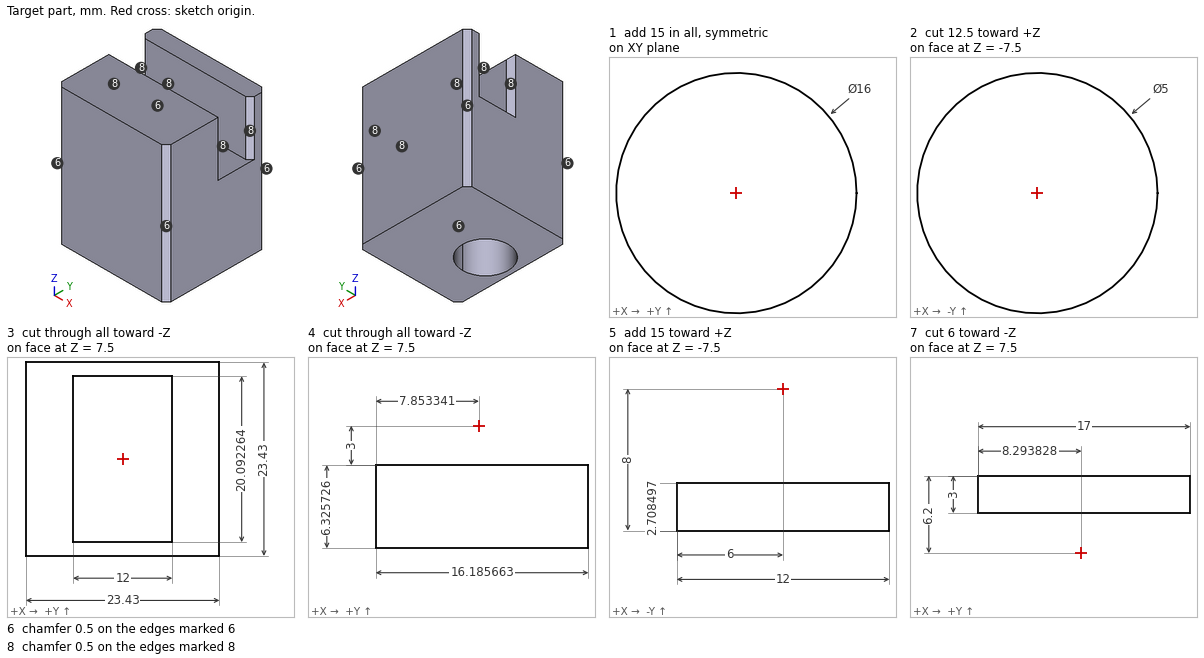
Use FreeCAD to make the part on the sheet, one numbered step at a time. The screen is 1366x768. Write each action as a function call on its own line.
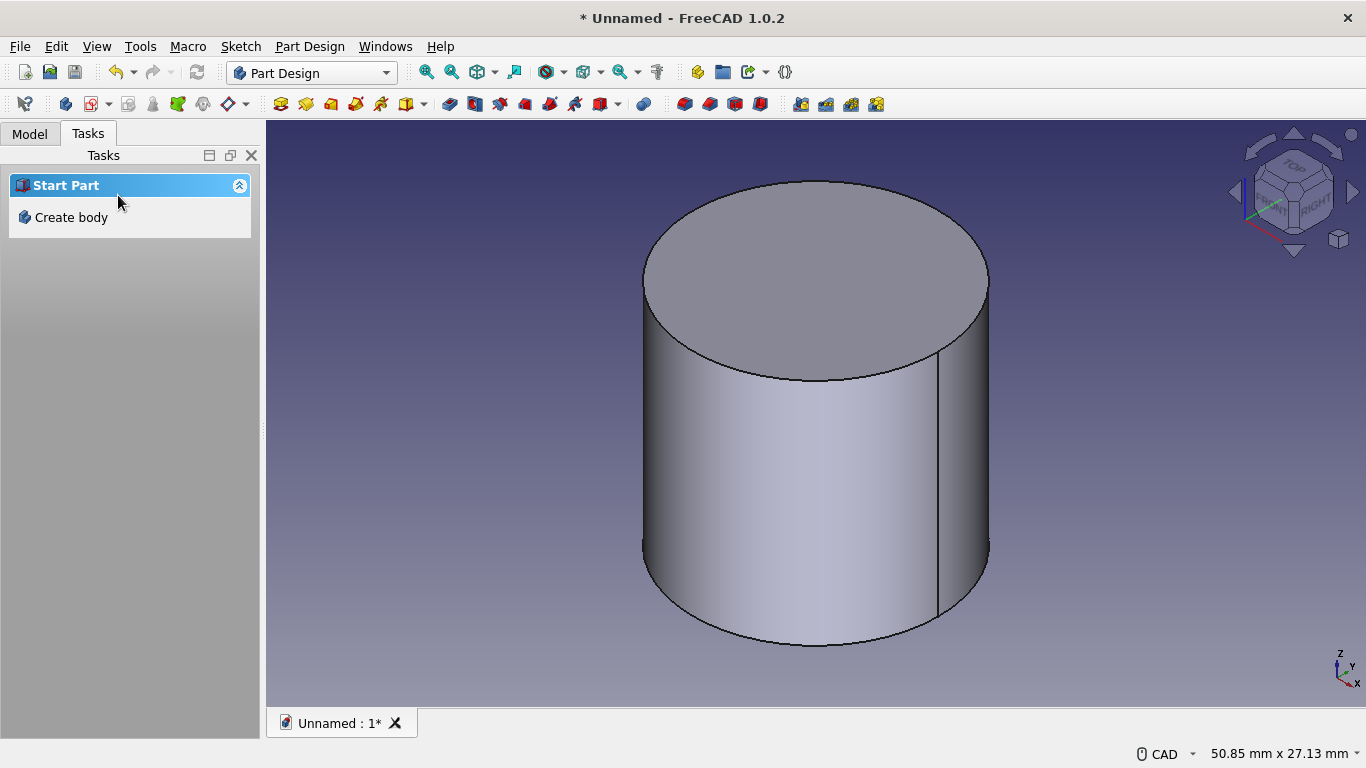
click(816, 280)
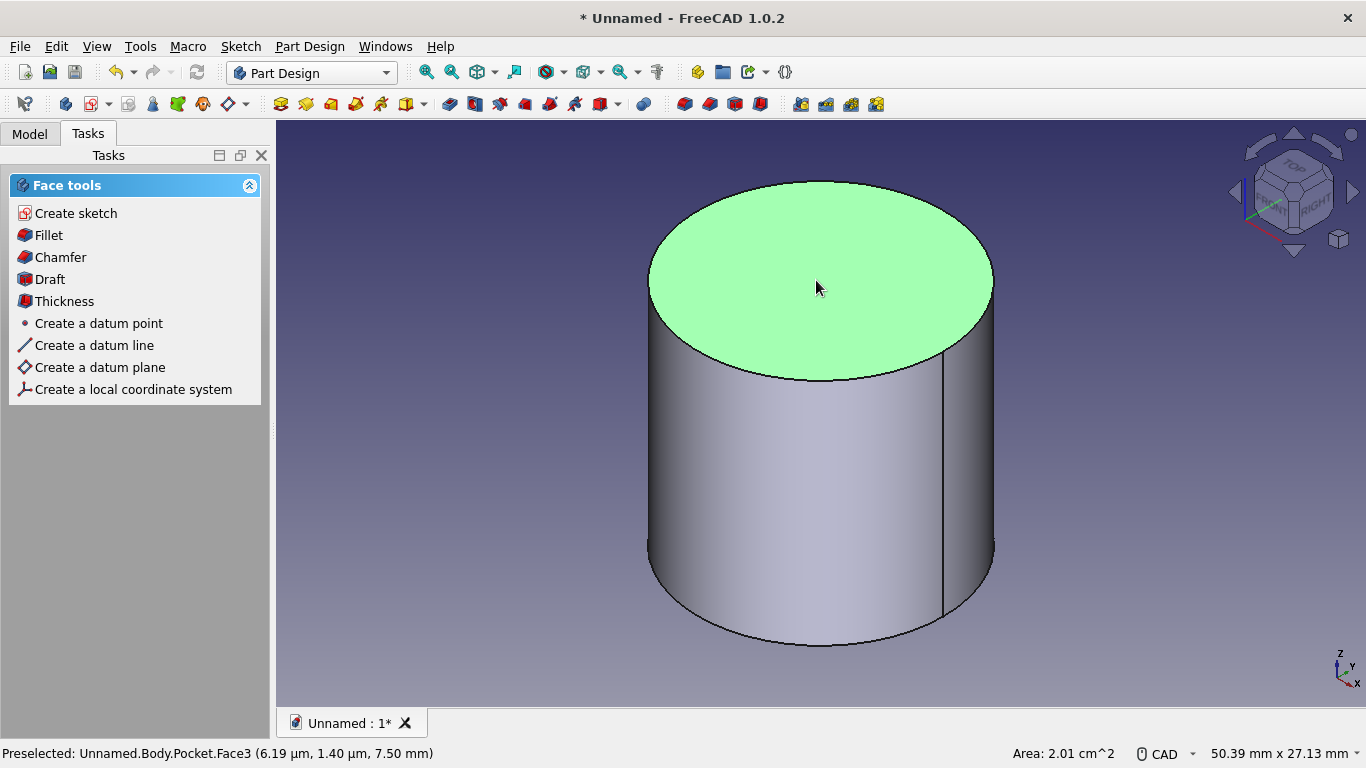
click(90, 104)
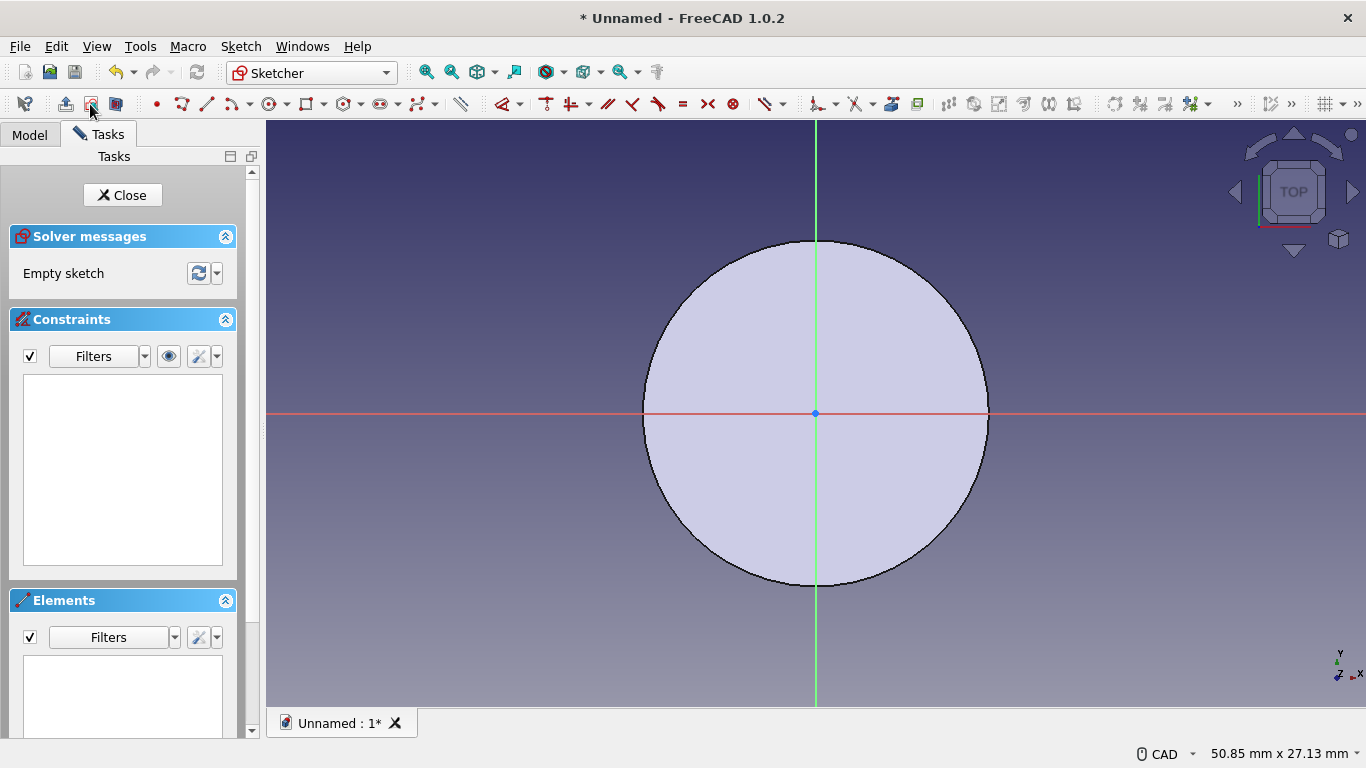
scroll(609, 414, down, 2)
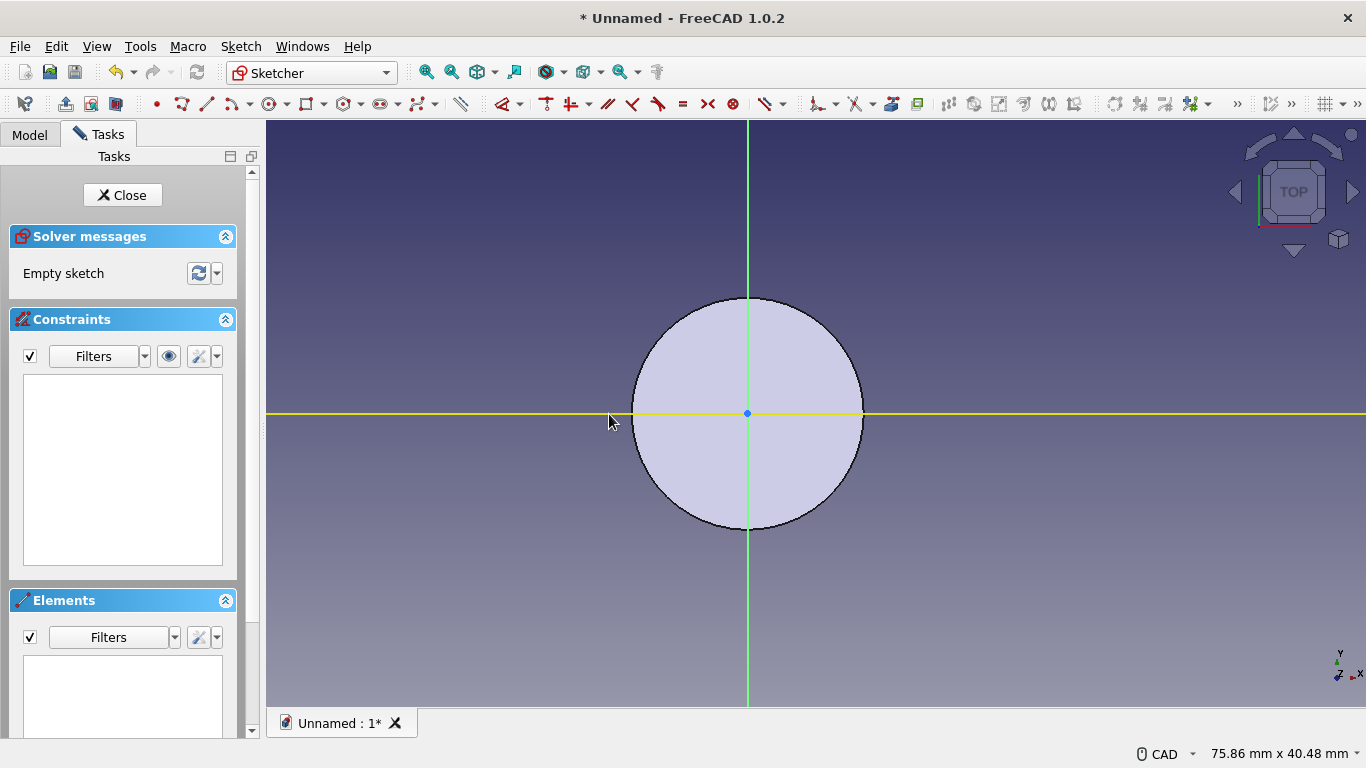
click(324, 104)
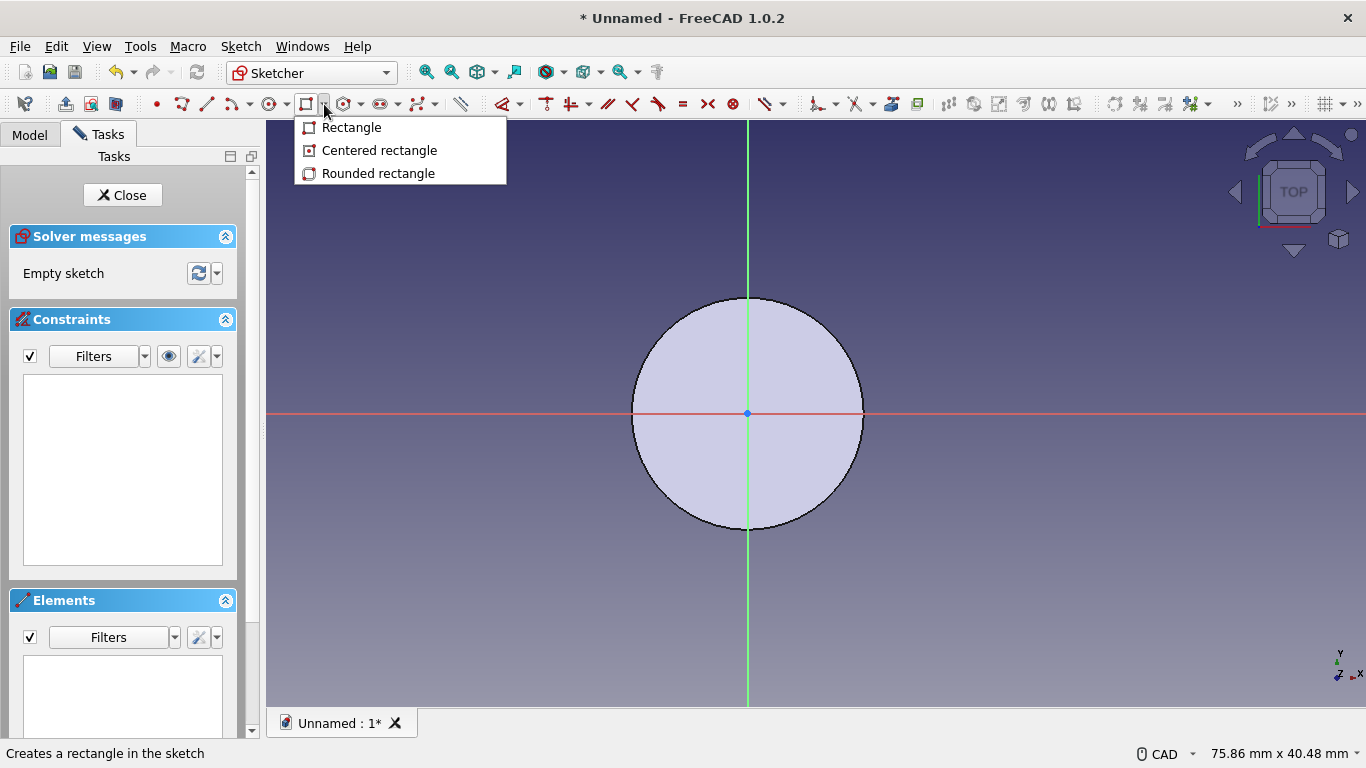
click(400, 150)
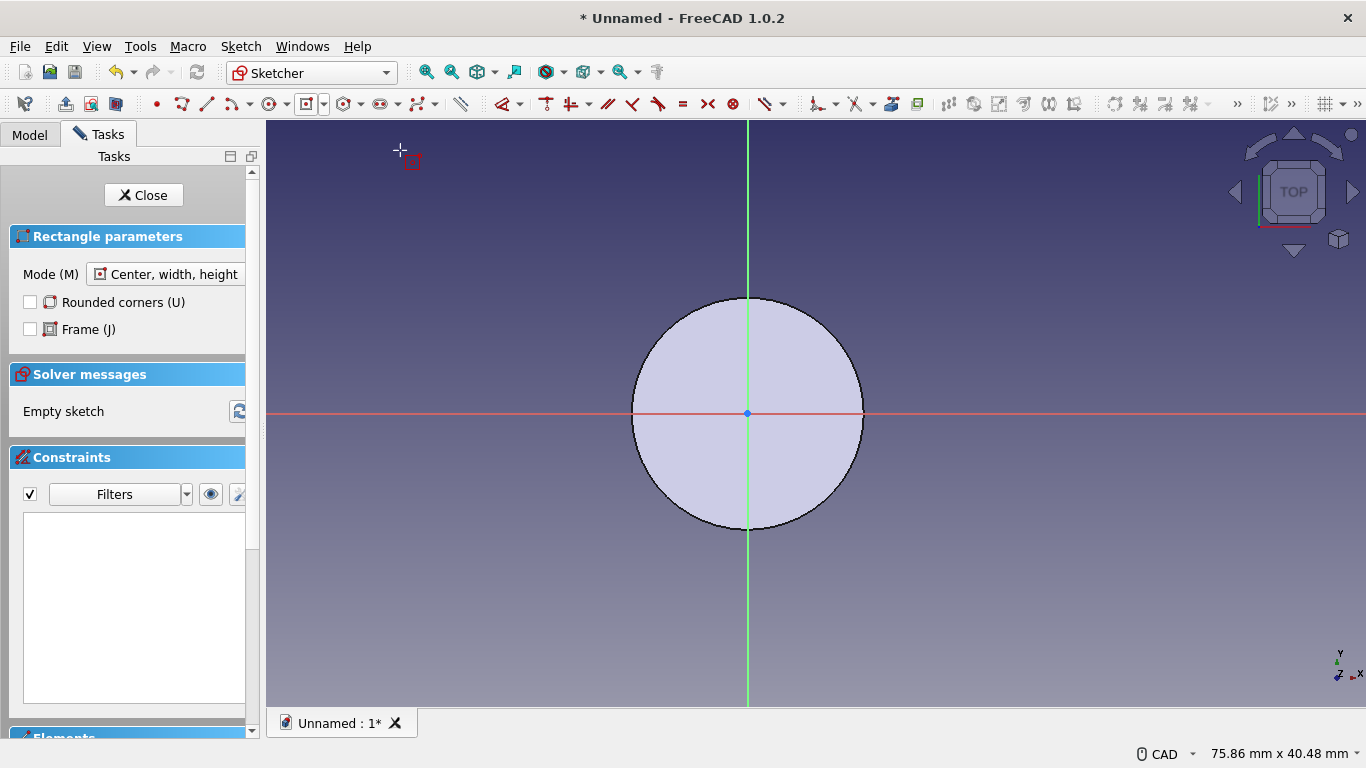
click(748, 414)
click(918, 244)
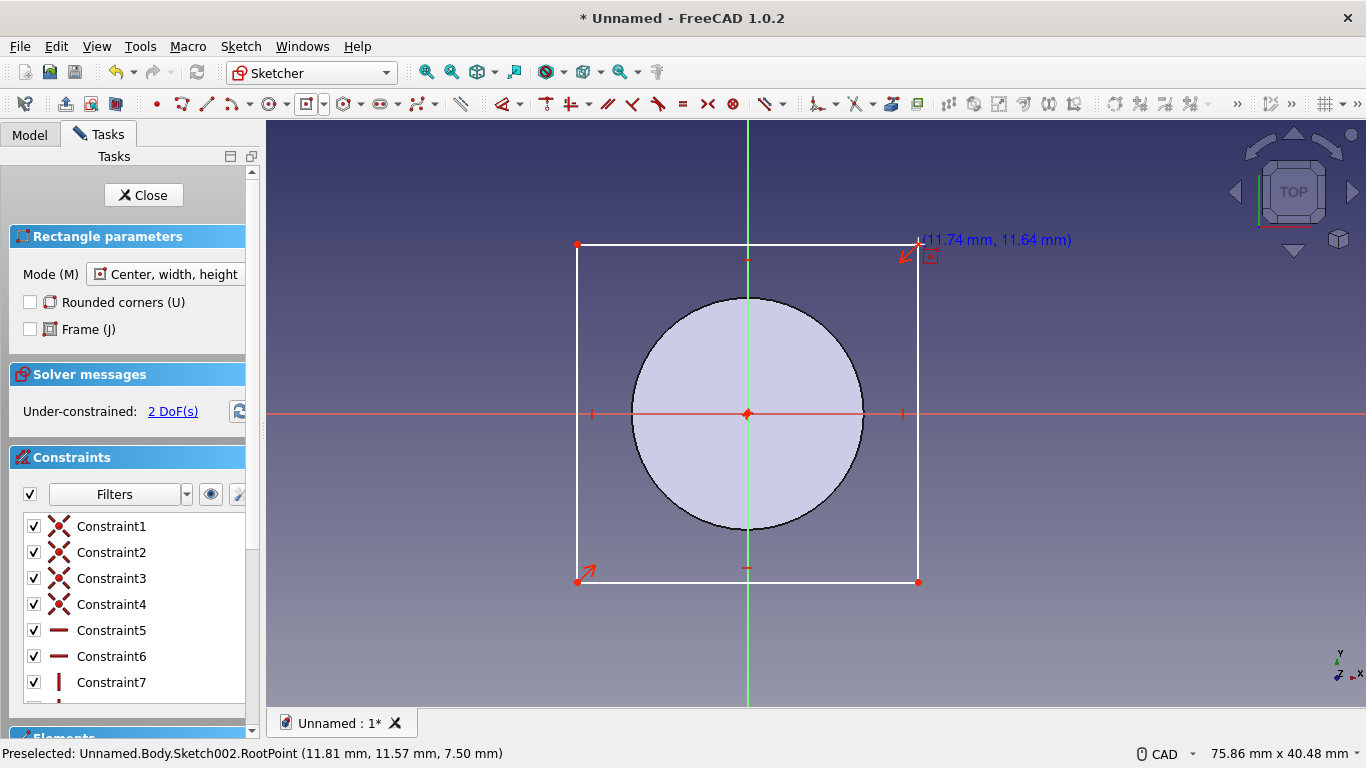
click(748, 414)
click(835, 268)
key(Escape)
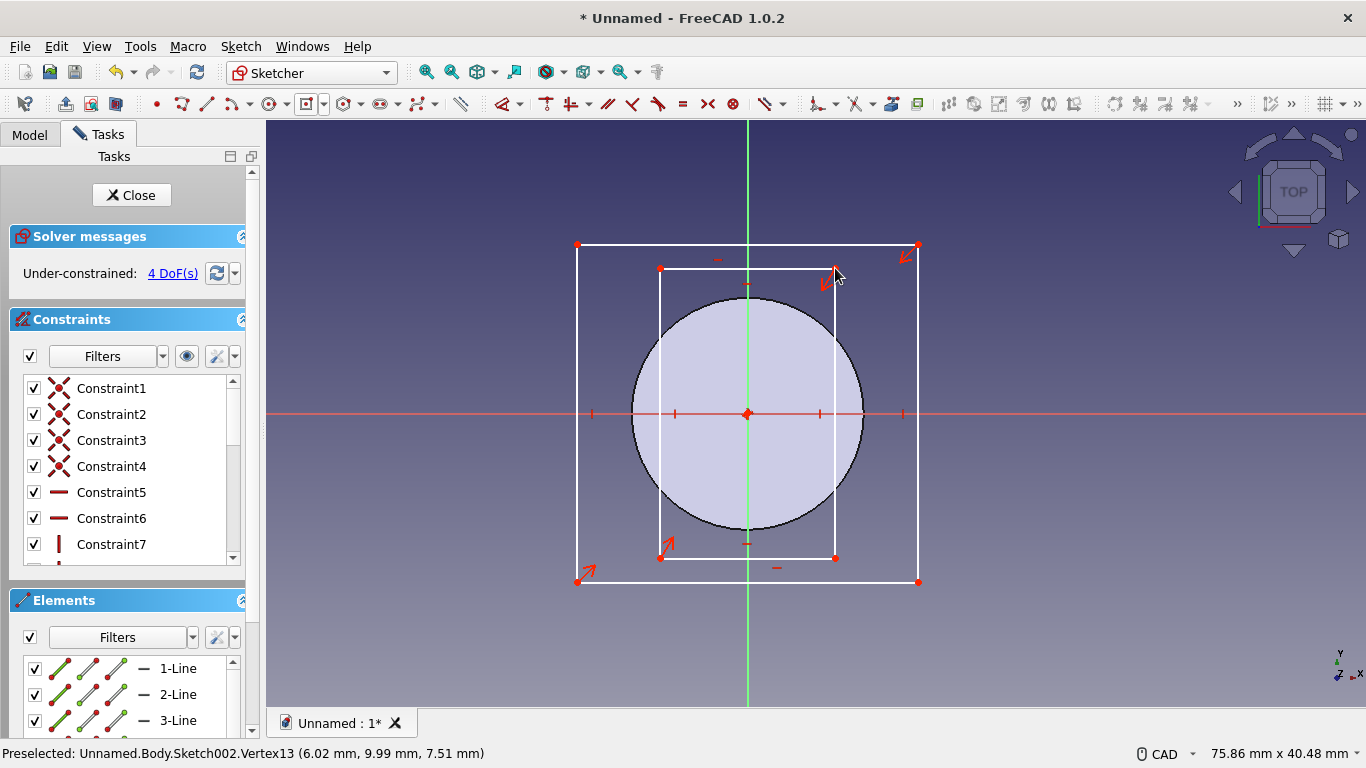
click(502, 104)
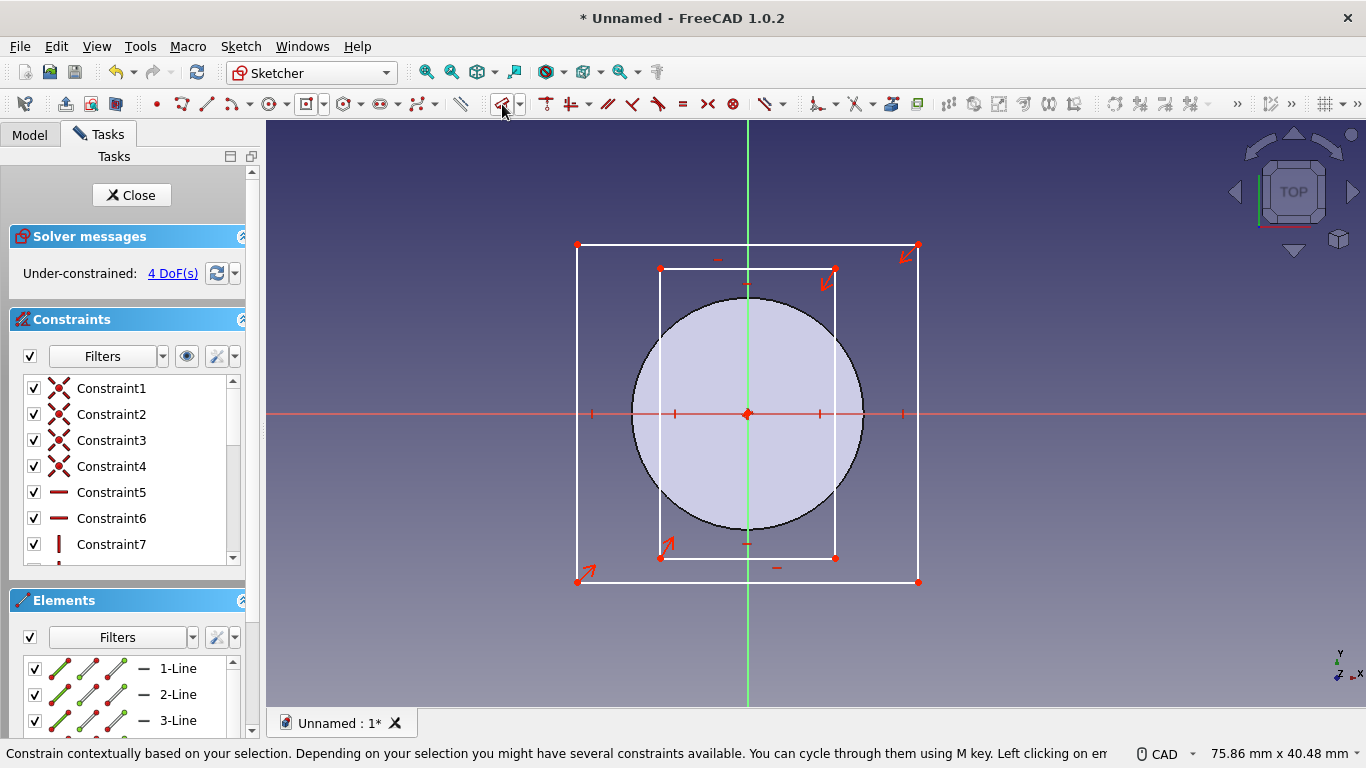
click(713, 559)
click(708, 525)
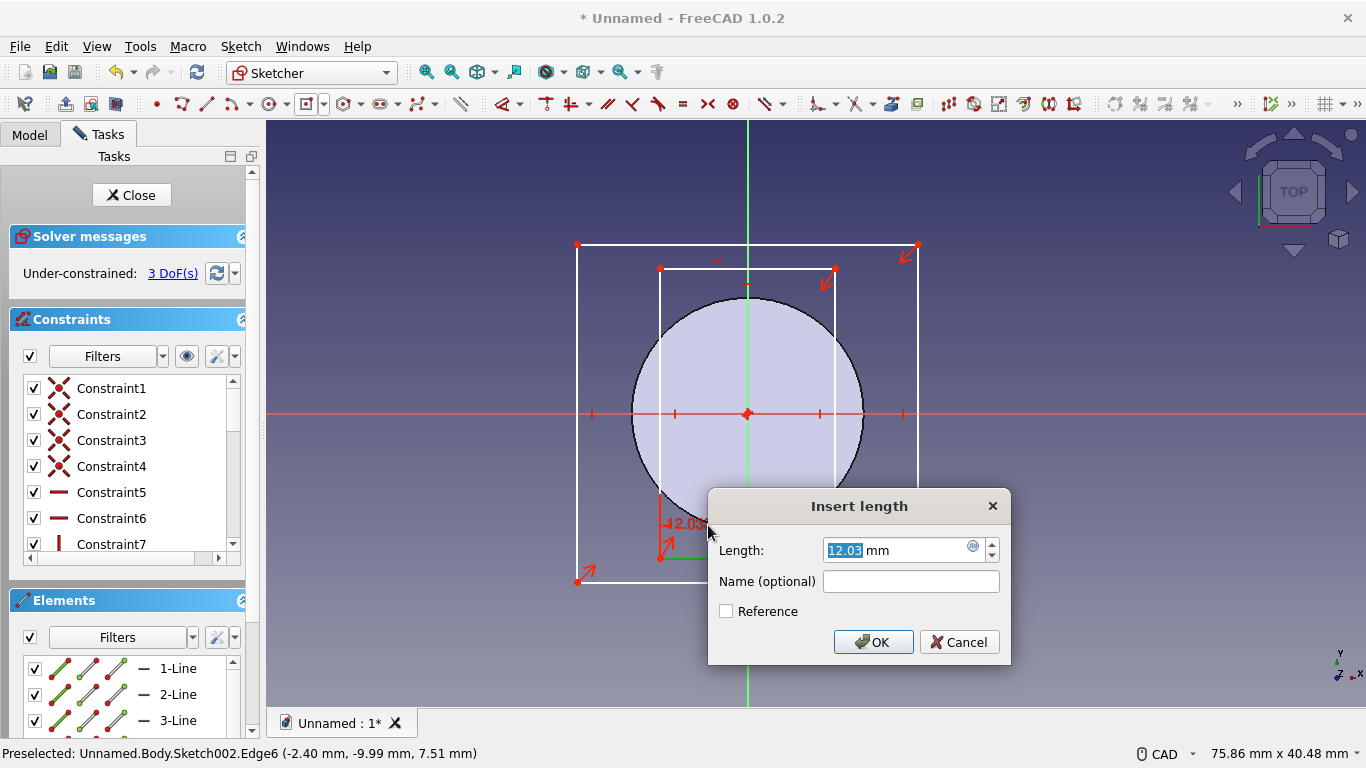
text(12)
key(Return)